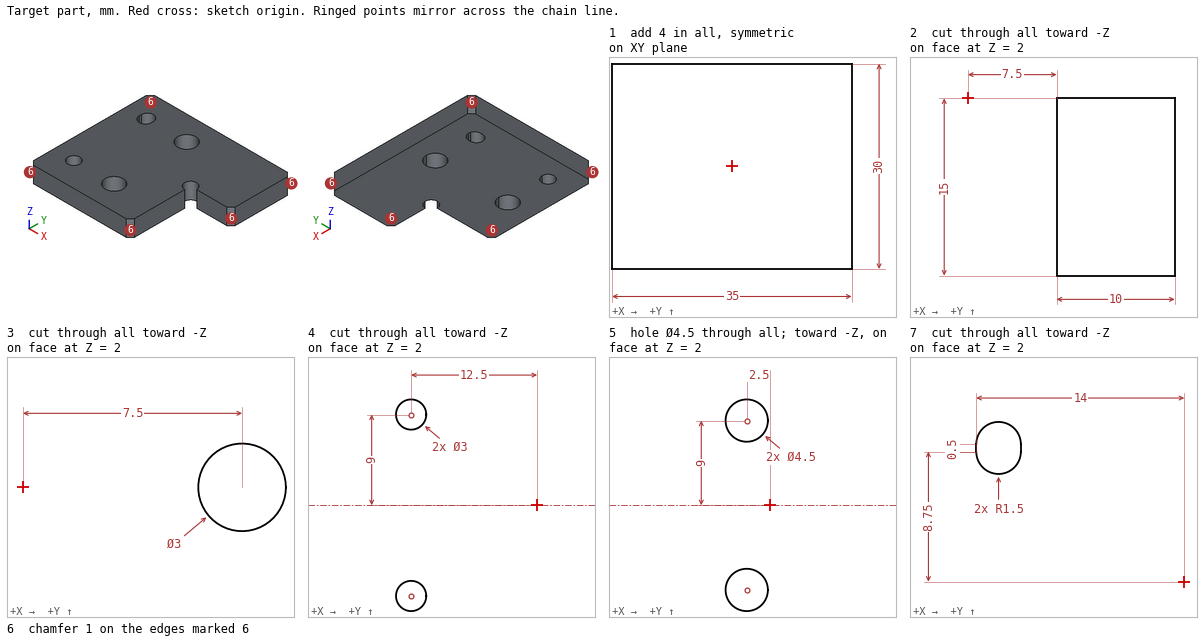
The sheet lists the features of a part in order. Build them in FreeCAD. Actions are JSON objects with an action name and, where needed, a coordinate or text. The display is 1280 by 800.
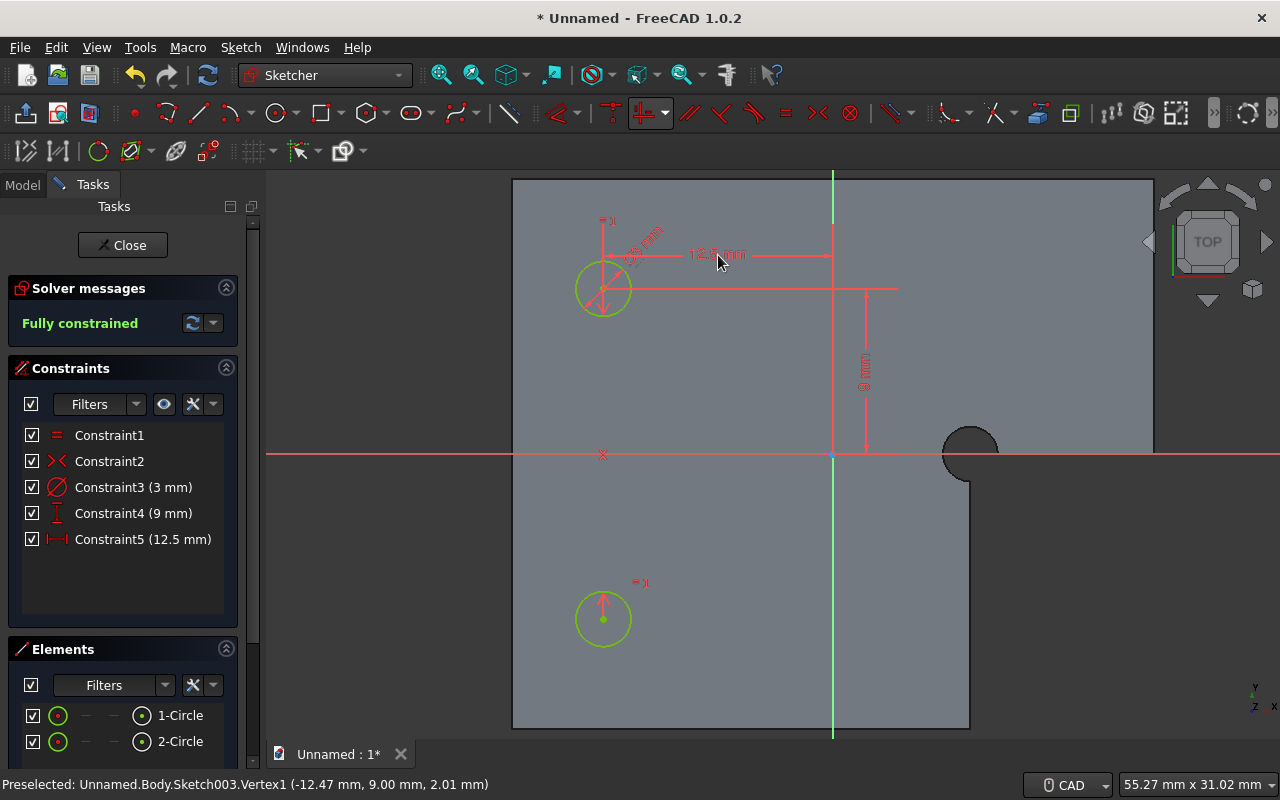
{"action": "left_click", "coordinate": [123, 245]}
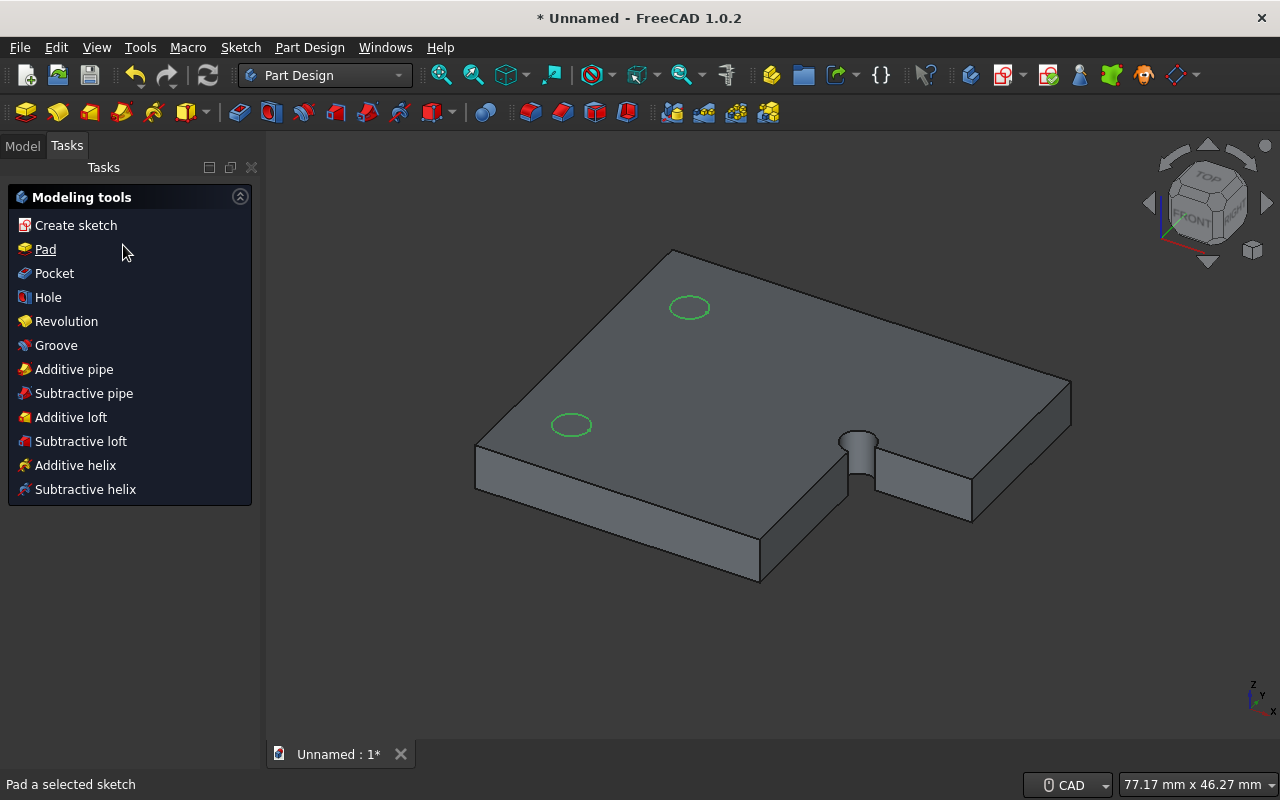
{"action": "left_click", "coordinate": [240, 112]}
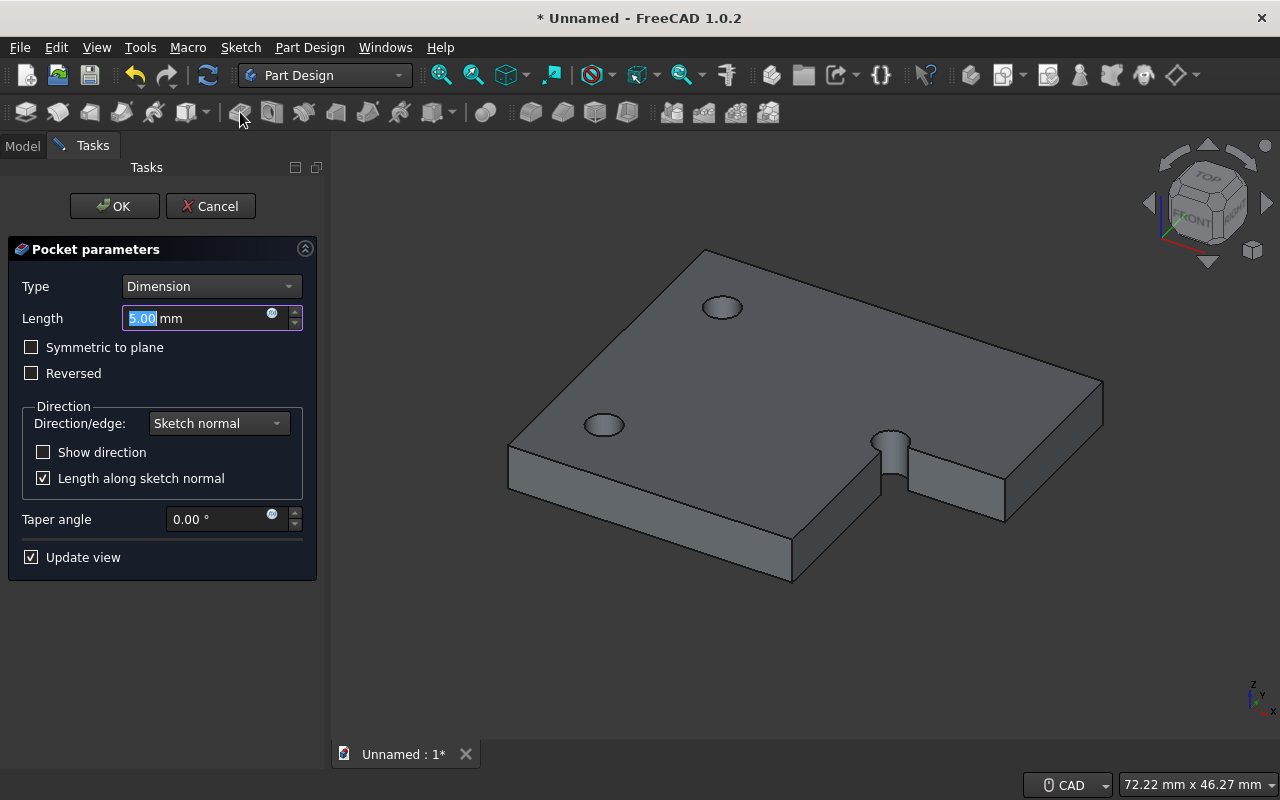
{"action": "left_click", "coordinate": [212, 286]}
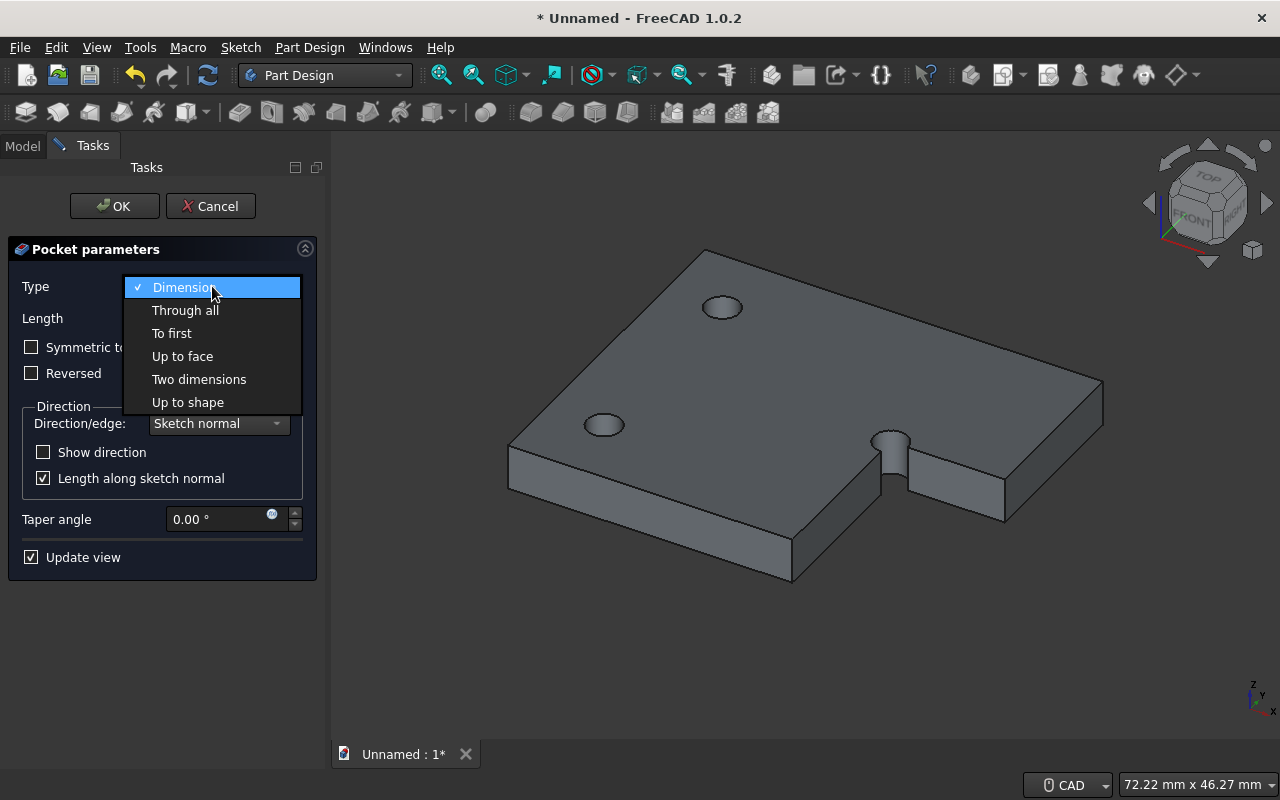
{"action": "left_click", "coordinate": [212, 310]}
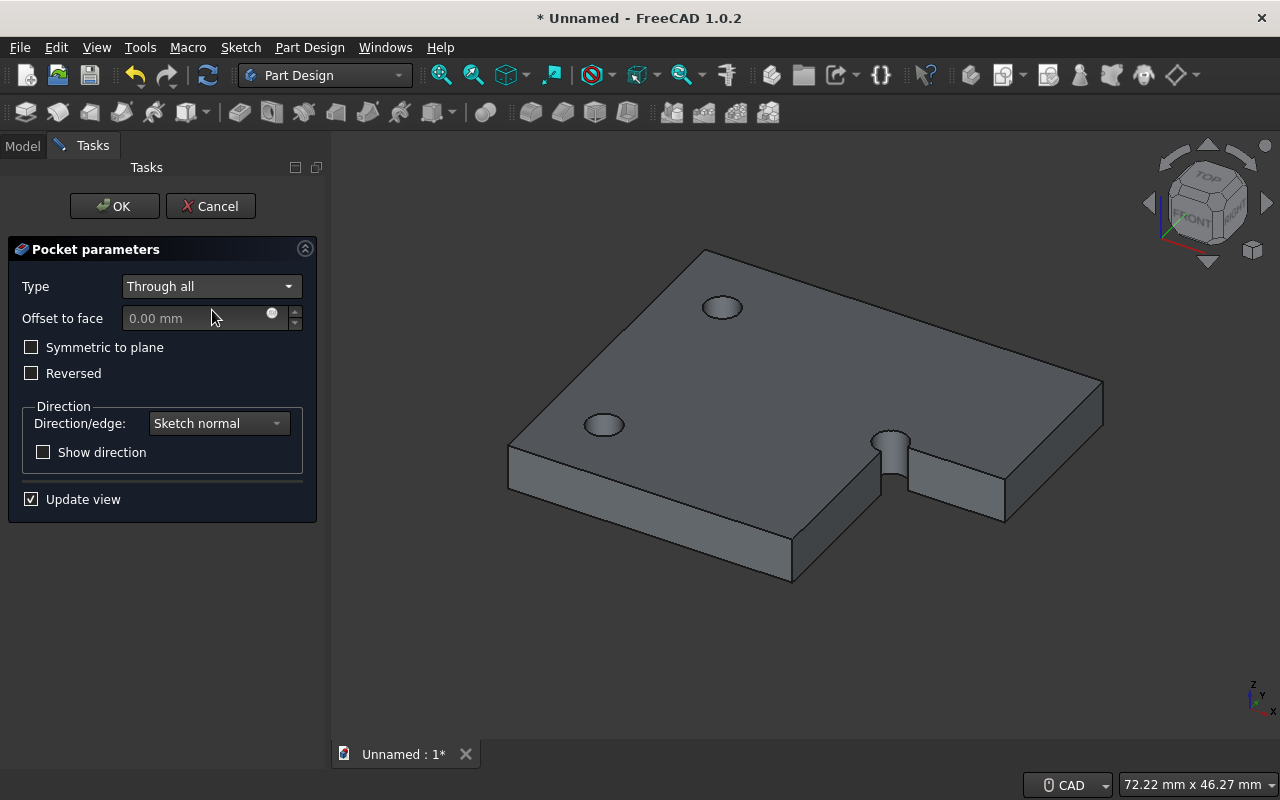
{"action": "left_click", "coordinate": [115, 206]}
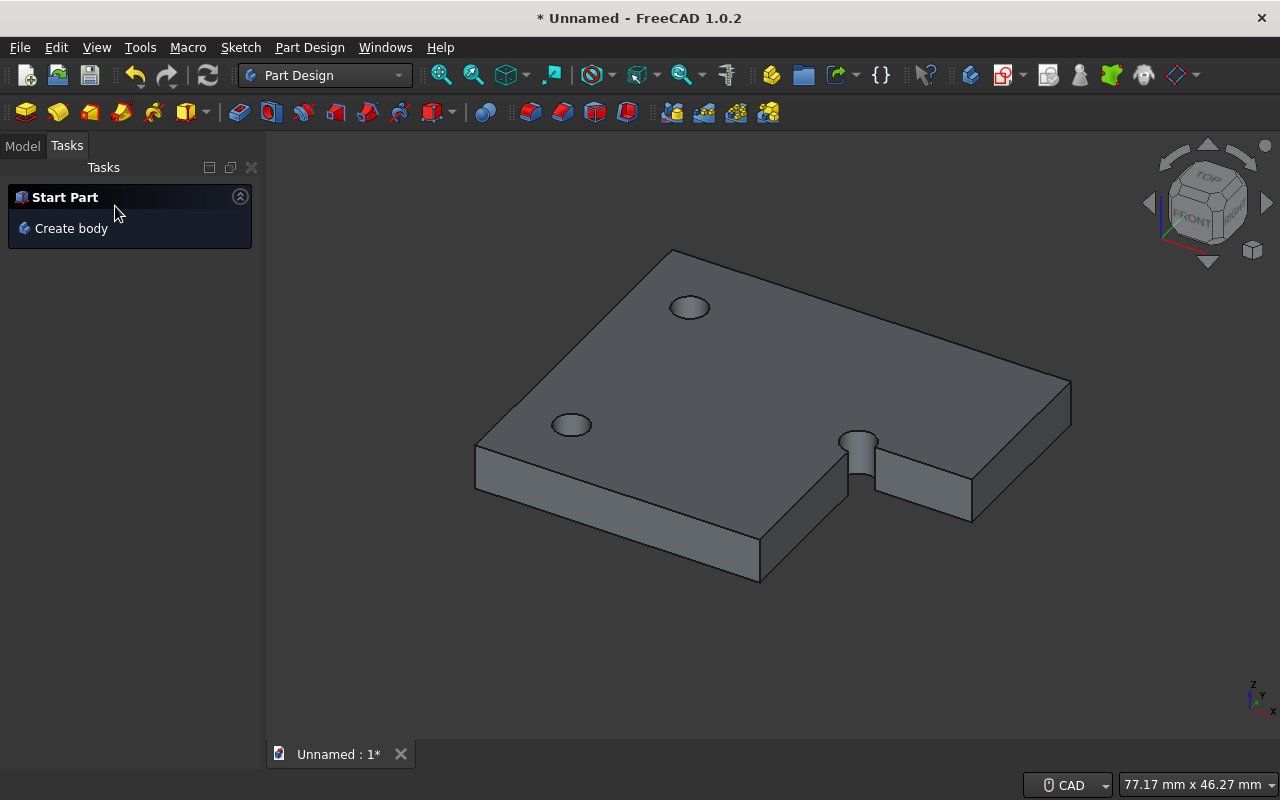
{"action": "left_click", "coordinate": [716, 394]}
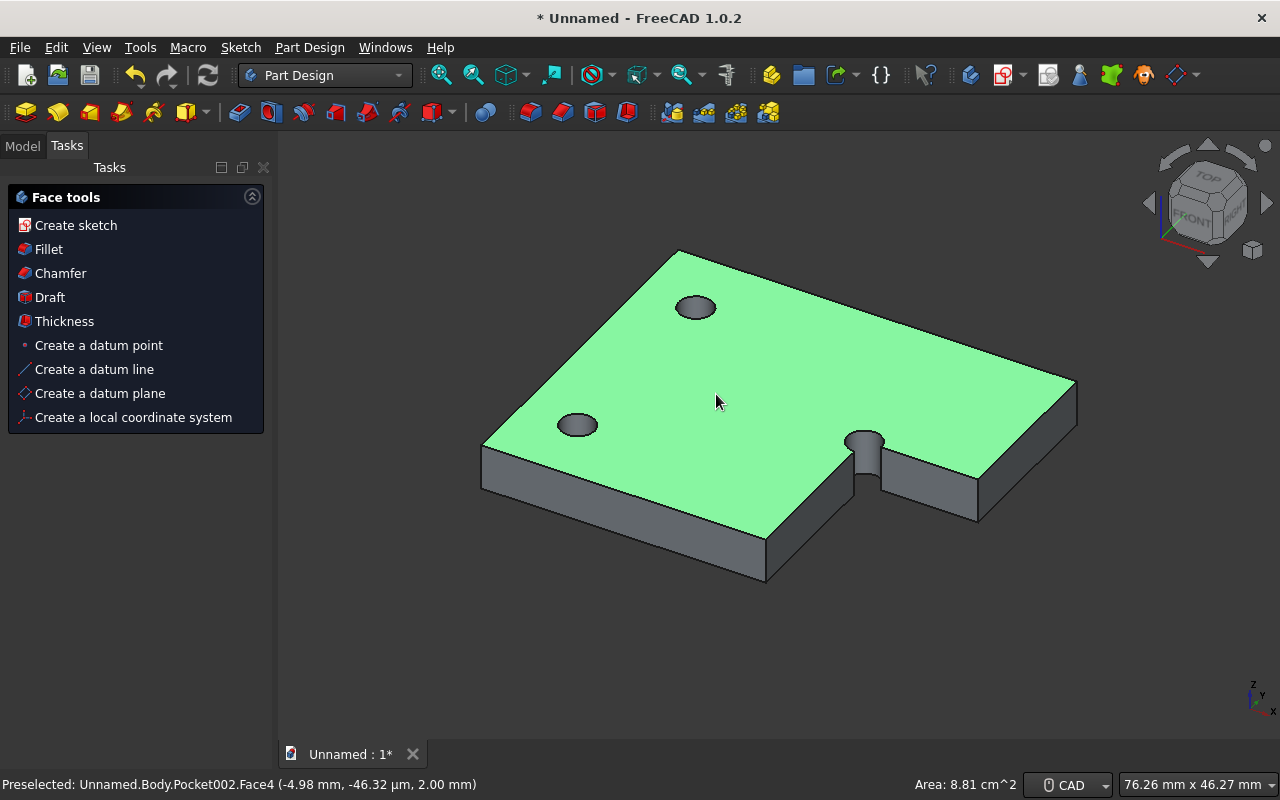
{"action": "left_click", "coordinate": [1004, 76]}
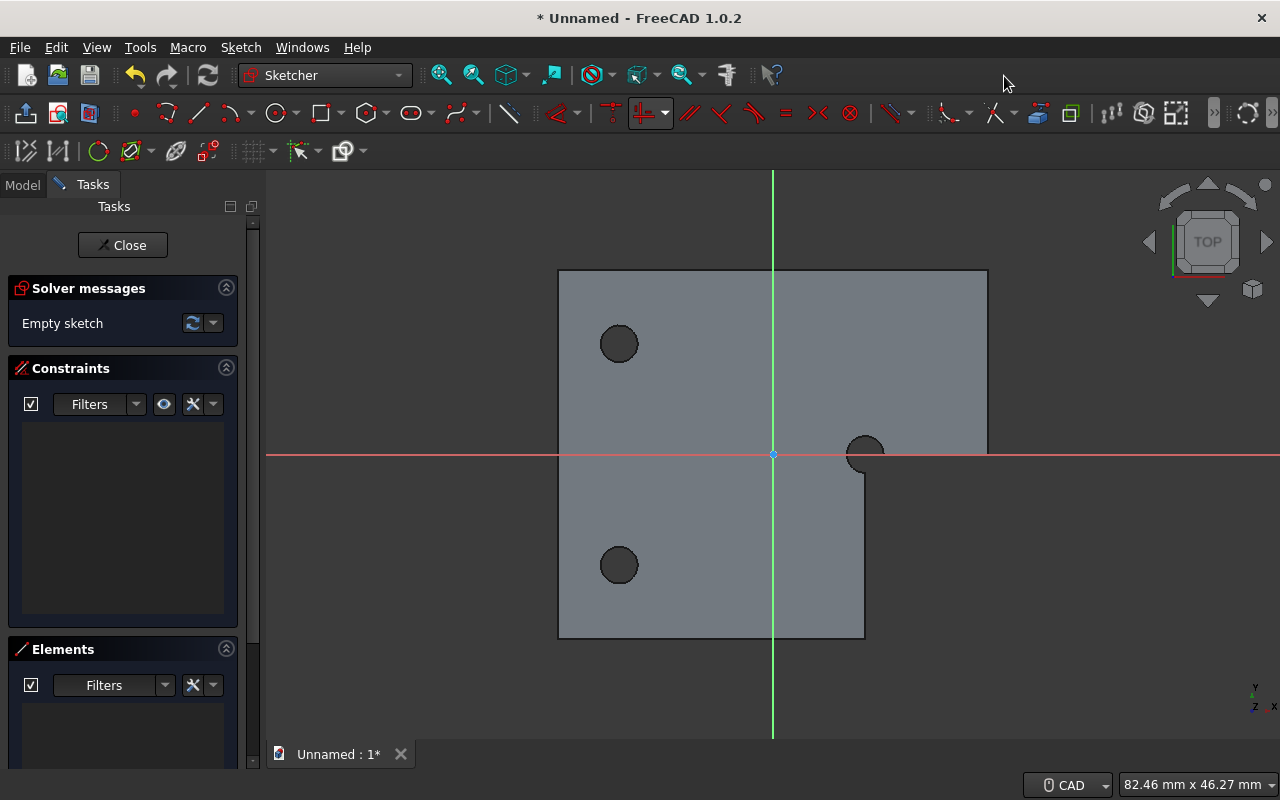
{"action": "key", "text": "g c"}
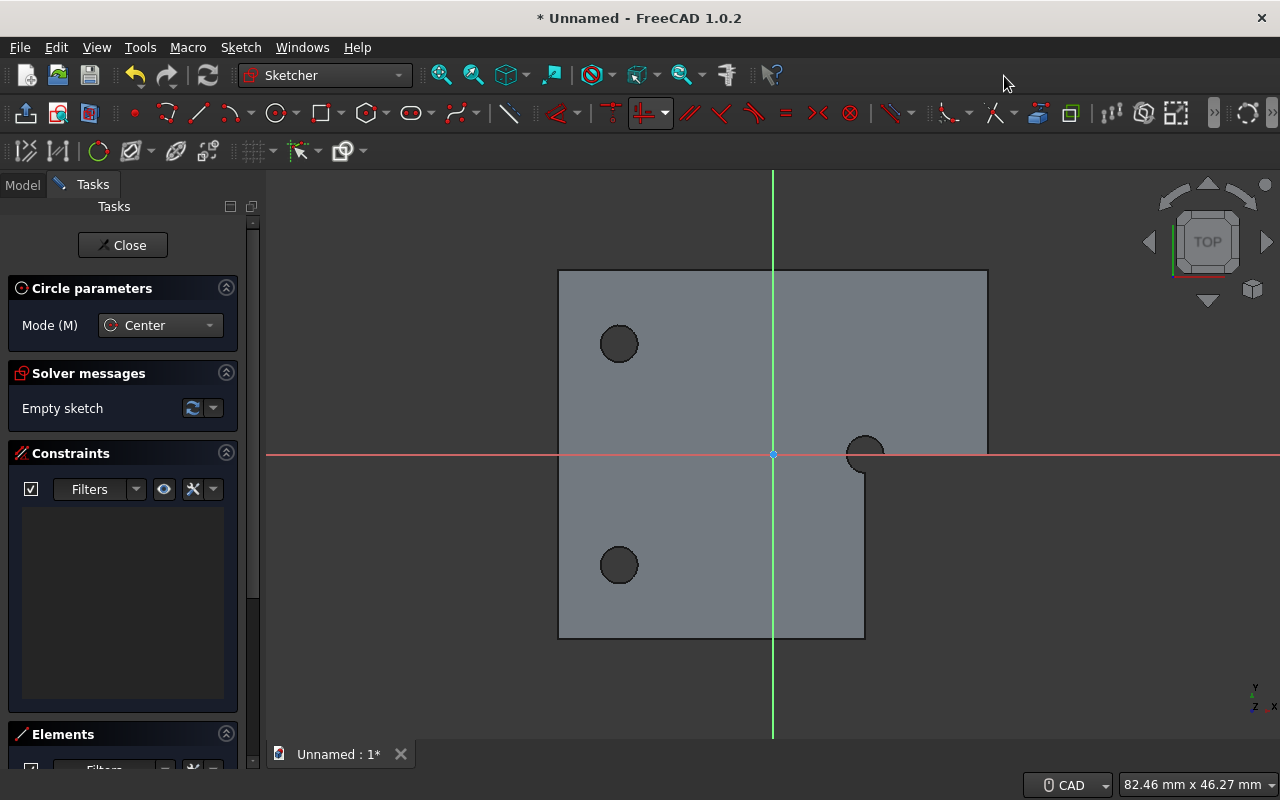
{"action": "left_click", "coordinate": [742, 344]}
{"action": "left_click", "coordinate": [723, 324]}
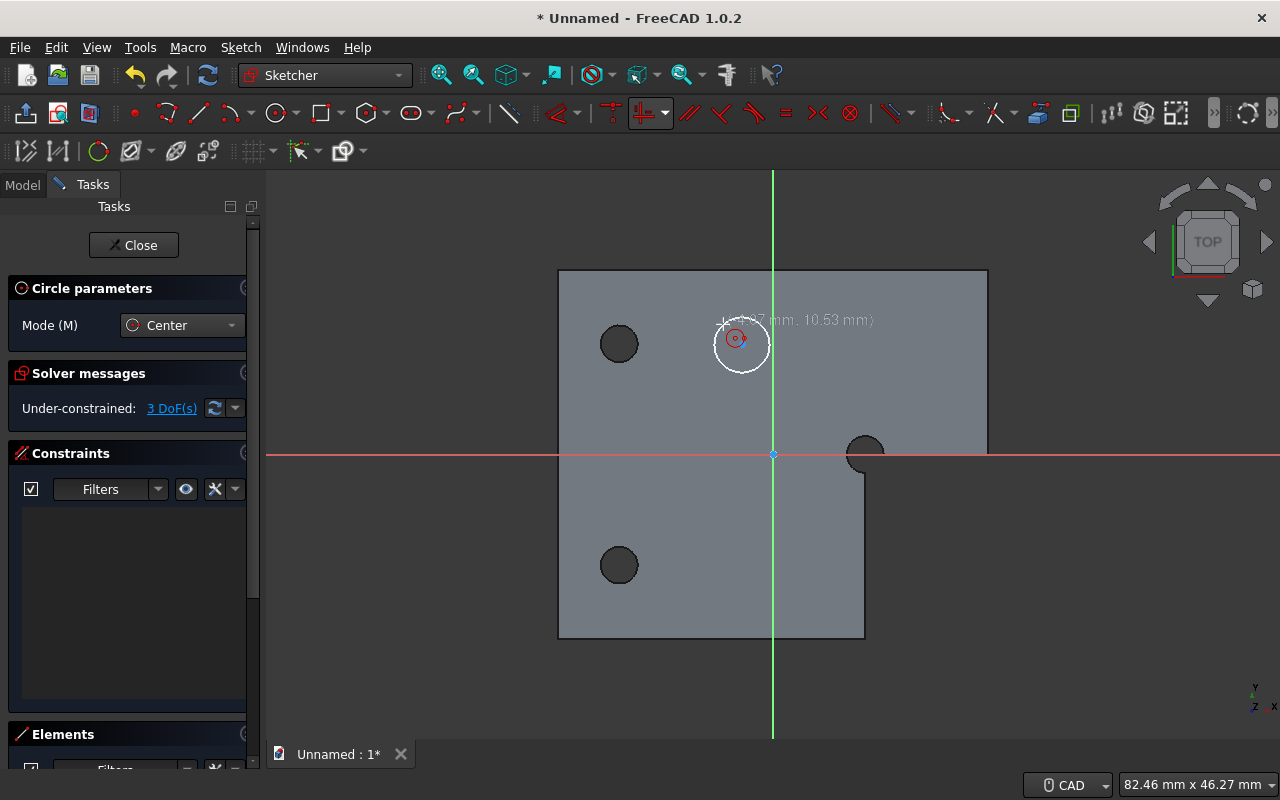
{"action": "left_click", "coordinate": [742, 565]}
{"action": "left_click", "coordinate": [723, 546]}
{"action": "key", "text": "Escape"}